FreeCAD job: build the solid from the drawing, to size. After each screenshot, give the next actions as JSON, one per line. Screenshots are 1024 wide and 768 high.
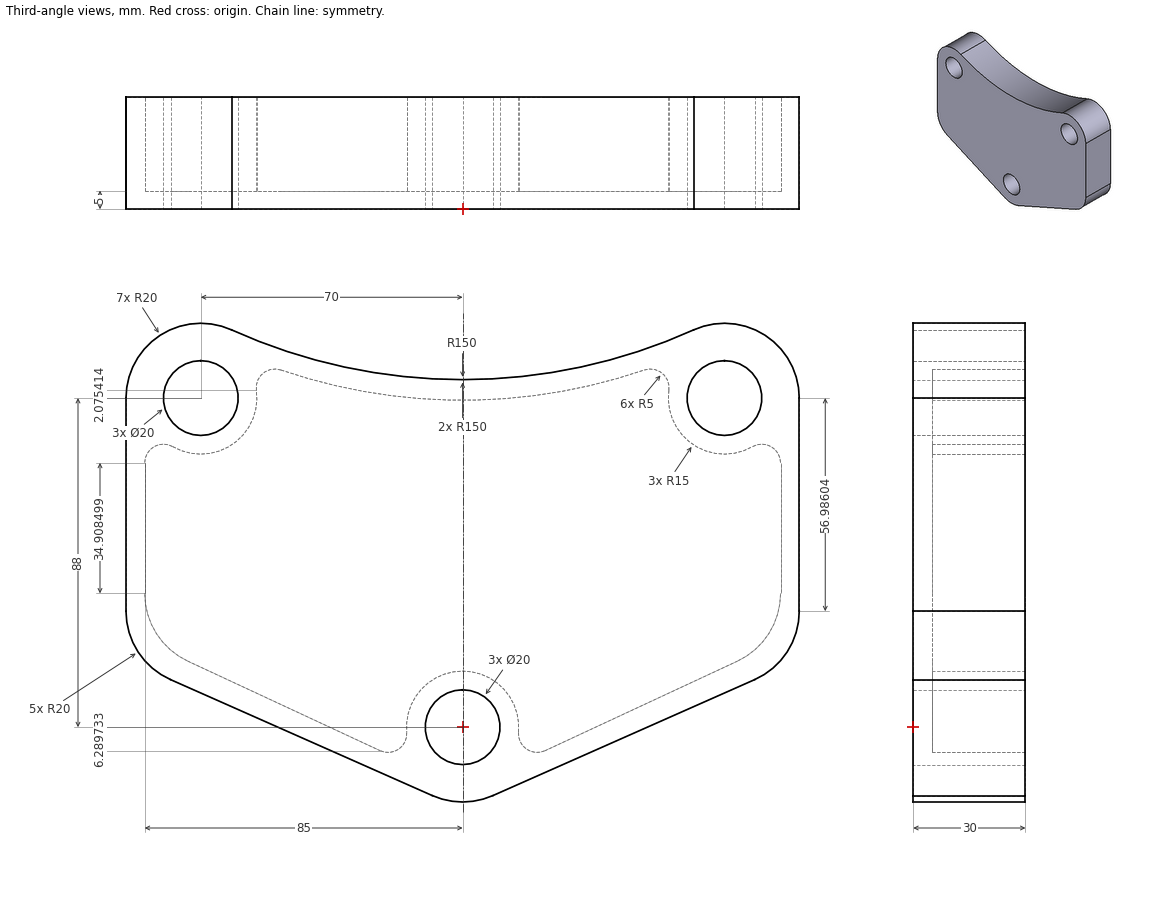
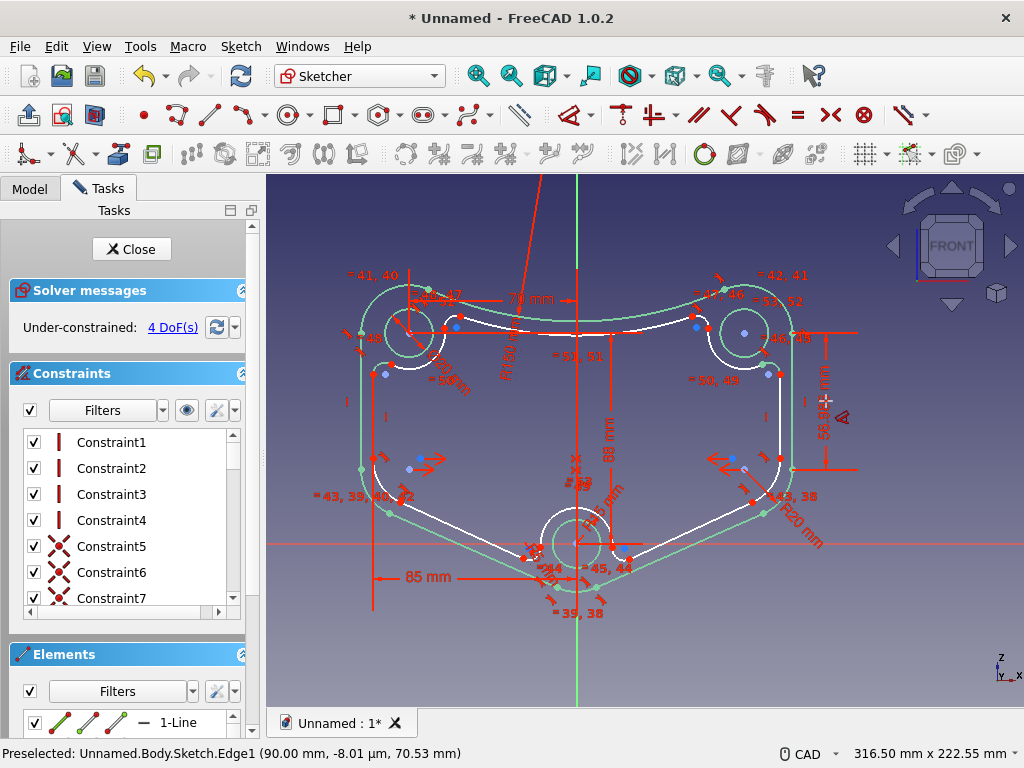
{"action": "left_click", "coordinate": [373, 400]}
{"action": "left_click", "coordinate": [339, 417]}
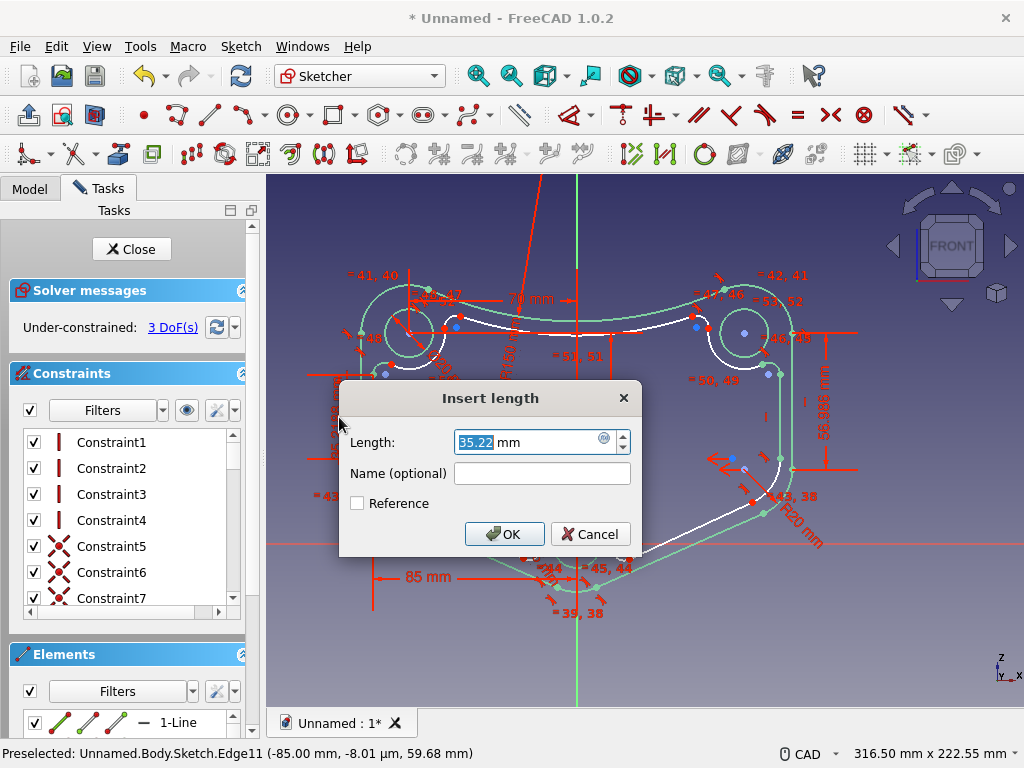
{"action": "type", "text": "34.908499"}
{"action": "key", "text": "Return"}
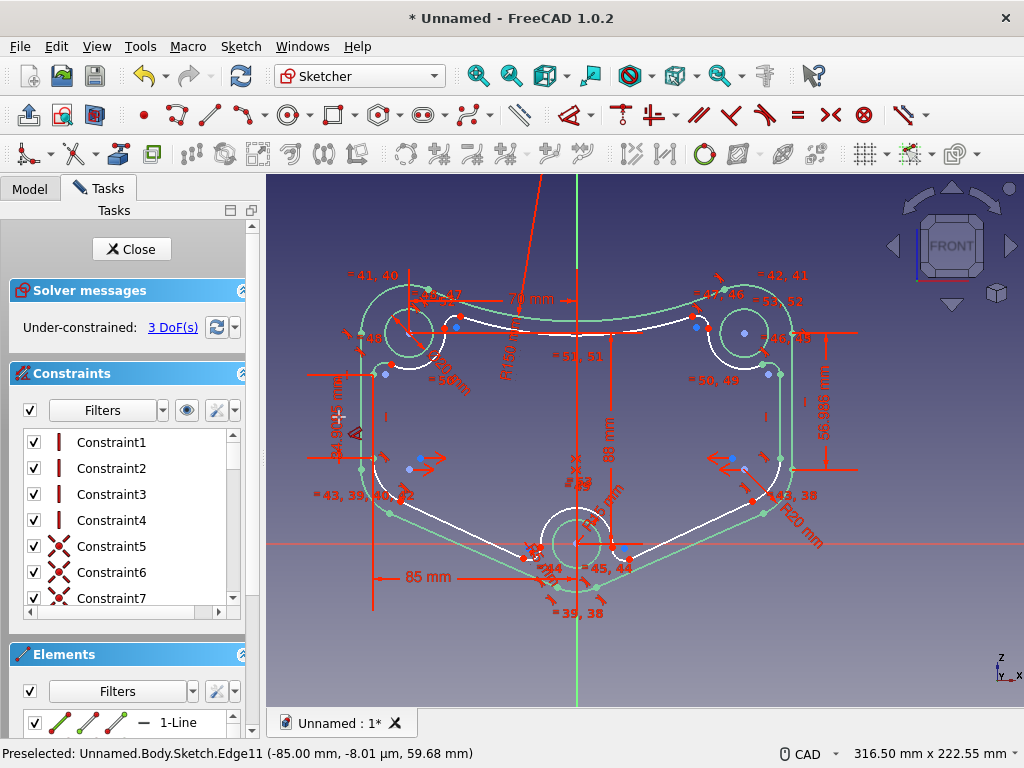
{"action": "scroll", "coordinate": [524, 559], "scroll_direction": "up", "scroll_amount": 5}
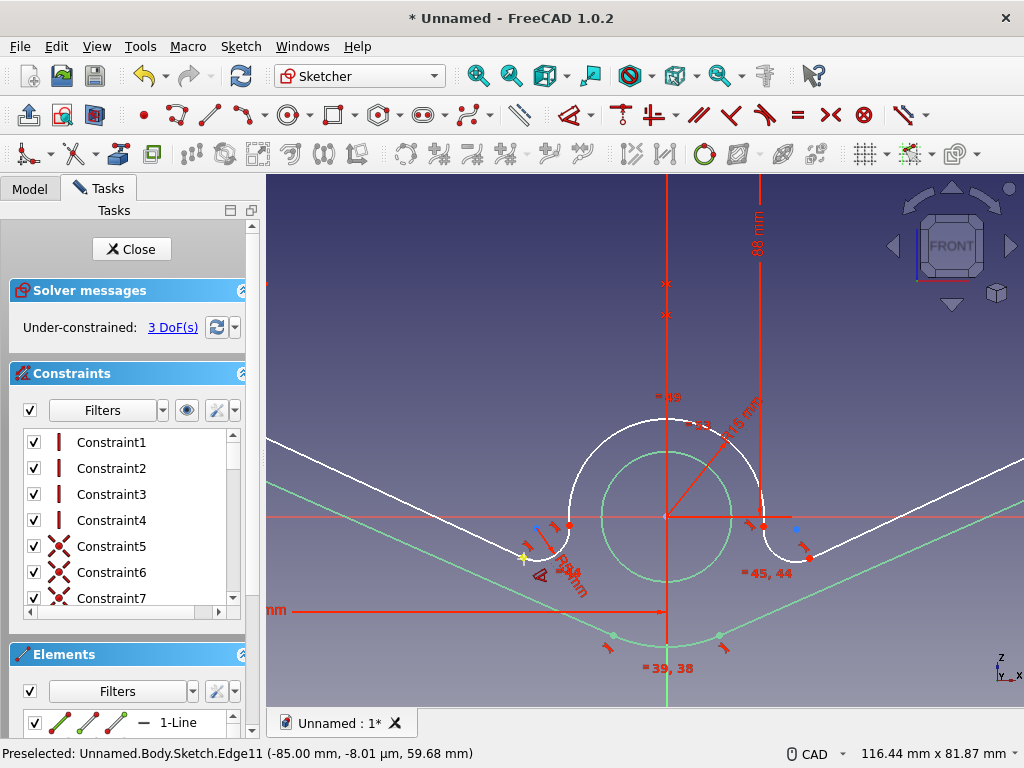
{"action": "left_click", "coordinate": [523, 558]}
{"action": "left_click", "coordinate": [701, 537]}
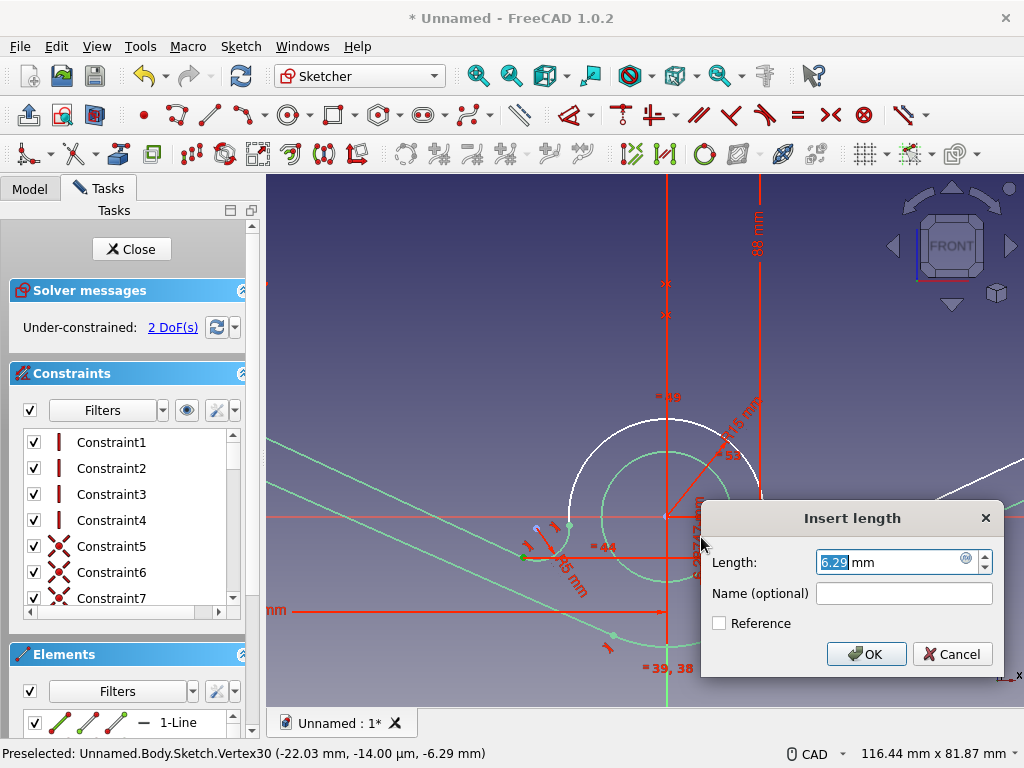
{"action": "type", "text": "6.289733"}
{"action": "key", "text": "Return"}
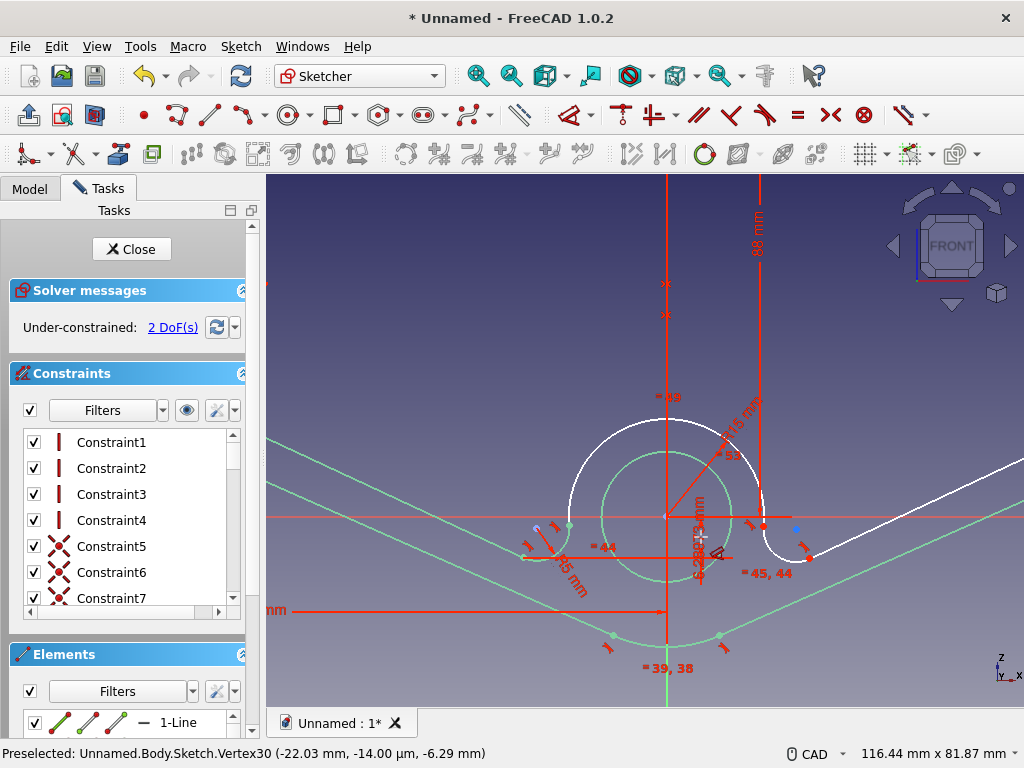
{"action": "left_click", "coordinate": [810, 559]}
{"action": "left_click", "coordinate": [585, 538]}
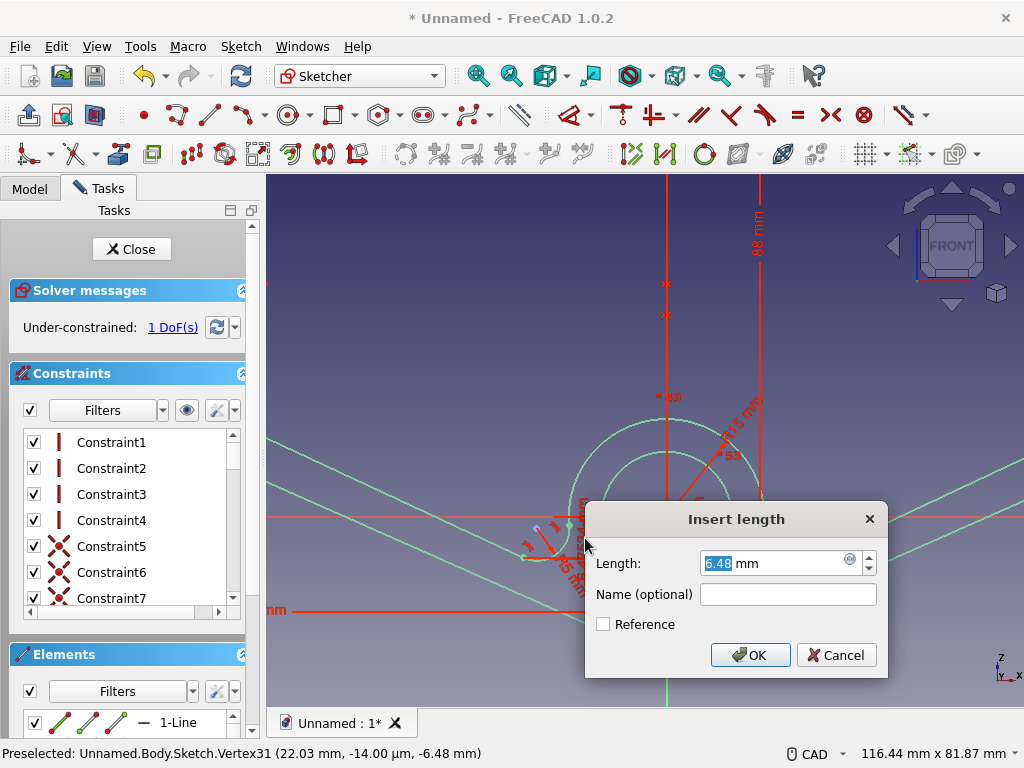
{"action": "type", "text": "6.289733"}
{"action": "key", "text": "Return"}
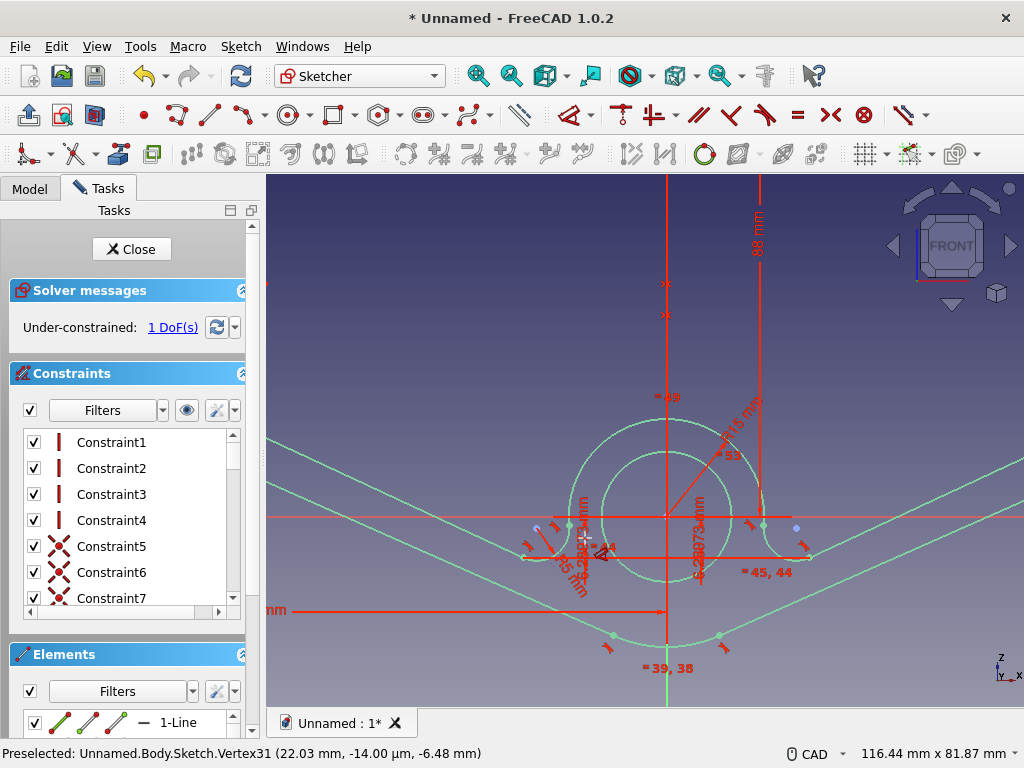
{"action": "scroll", "coordinate": [524, 559], "scroll_direction": "down", "scroll_amount": 5}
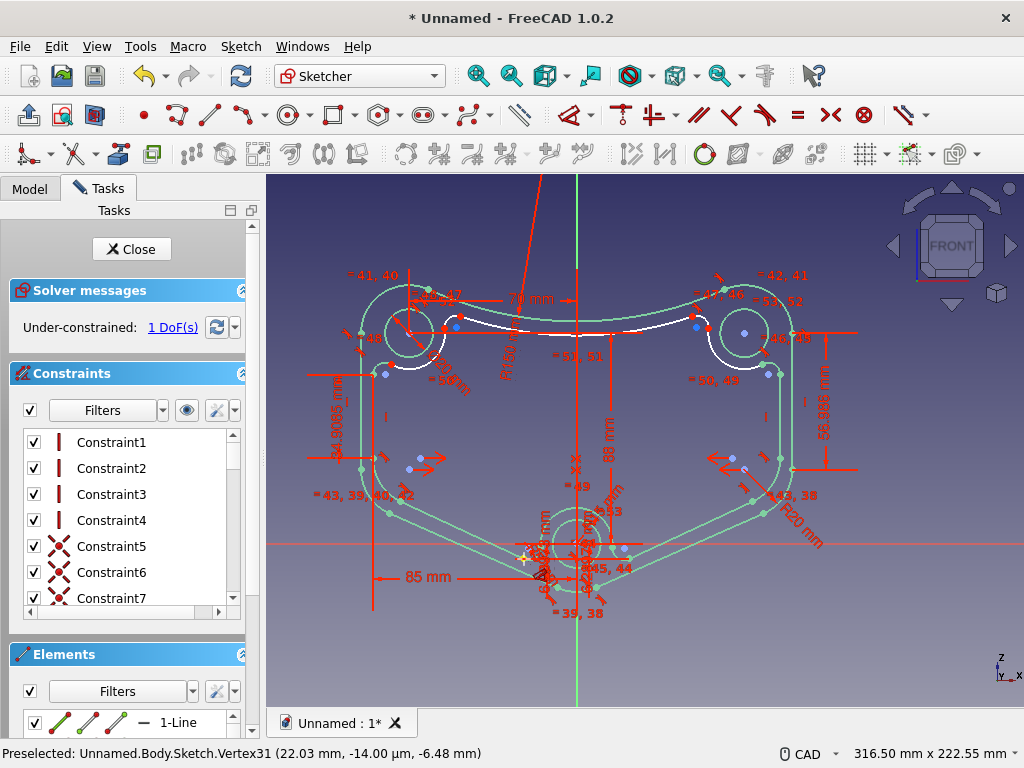
{"action": "scroll", "coordinate": [445, 329], "scroll_direction": "up", "scroll_amount": 11}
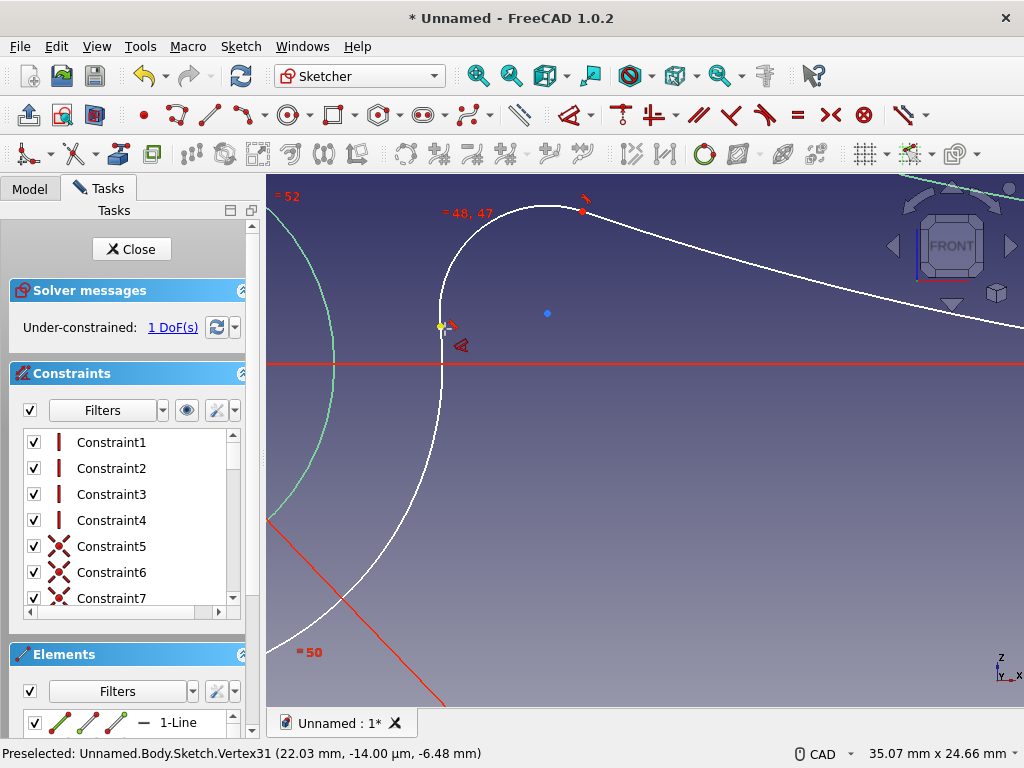
{"action": "left_click", "coordinate": [440, 326]}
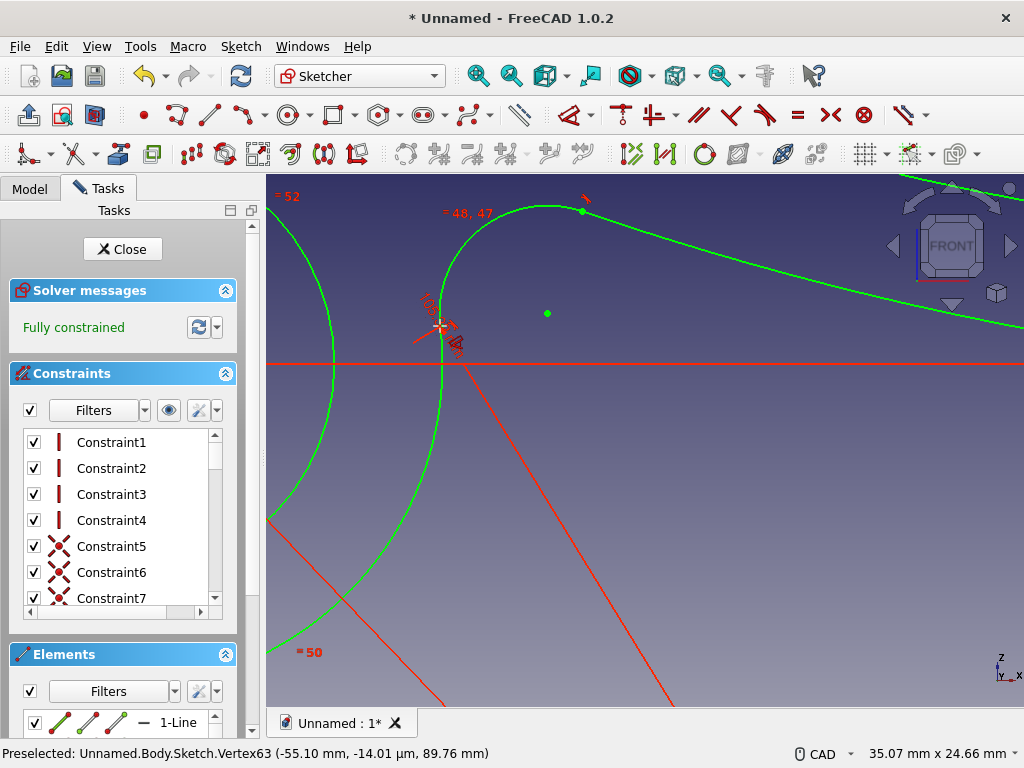
{"action": "scroll", "coordinate": [445, 329], "scroll_direction": "down", "scroll_amount": 11}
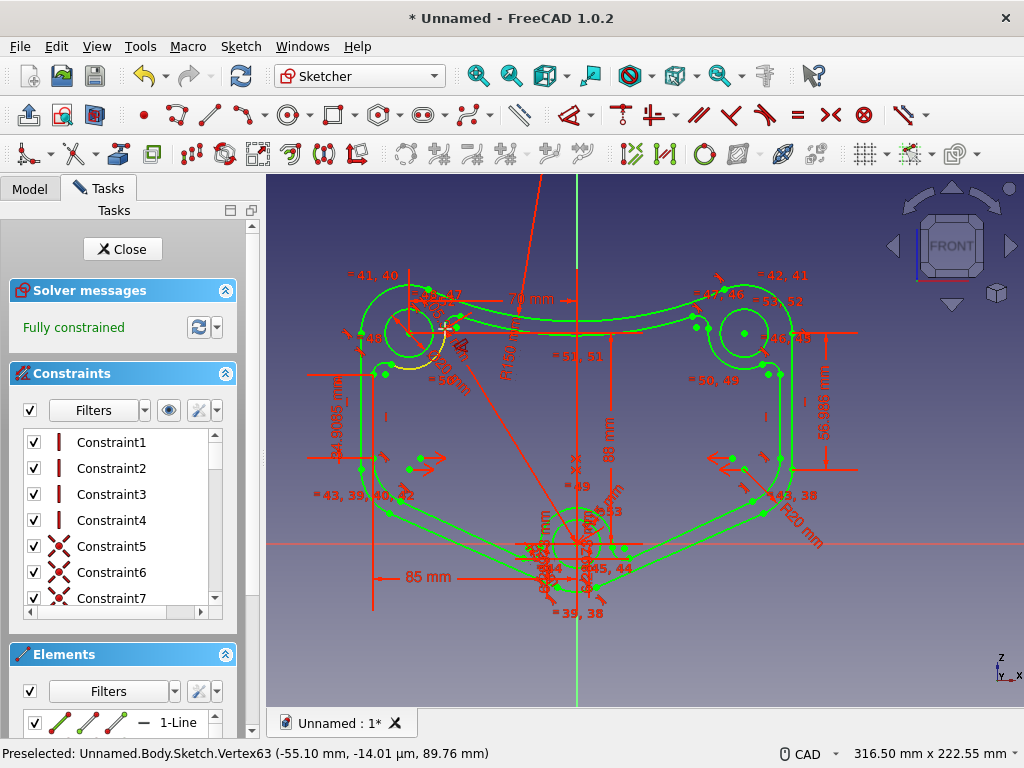
{"action": "scroll", "coordinate": [409, 333], "scroll_direction": "up", "scroll_amount": 11}